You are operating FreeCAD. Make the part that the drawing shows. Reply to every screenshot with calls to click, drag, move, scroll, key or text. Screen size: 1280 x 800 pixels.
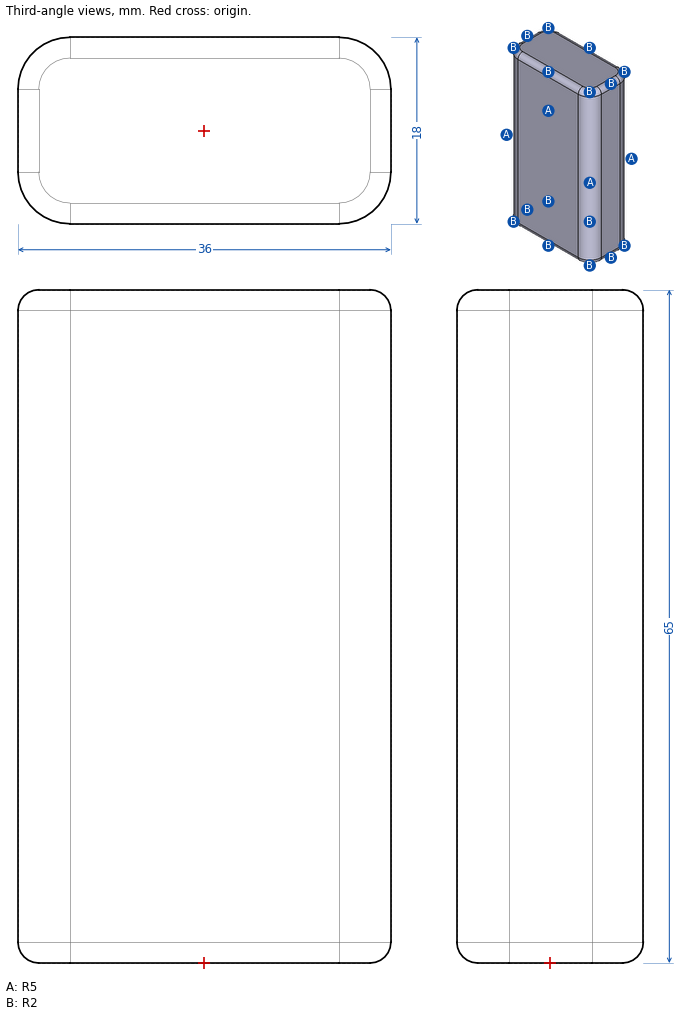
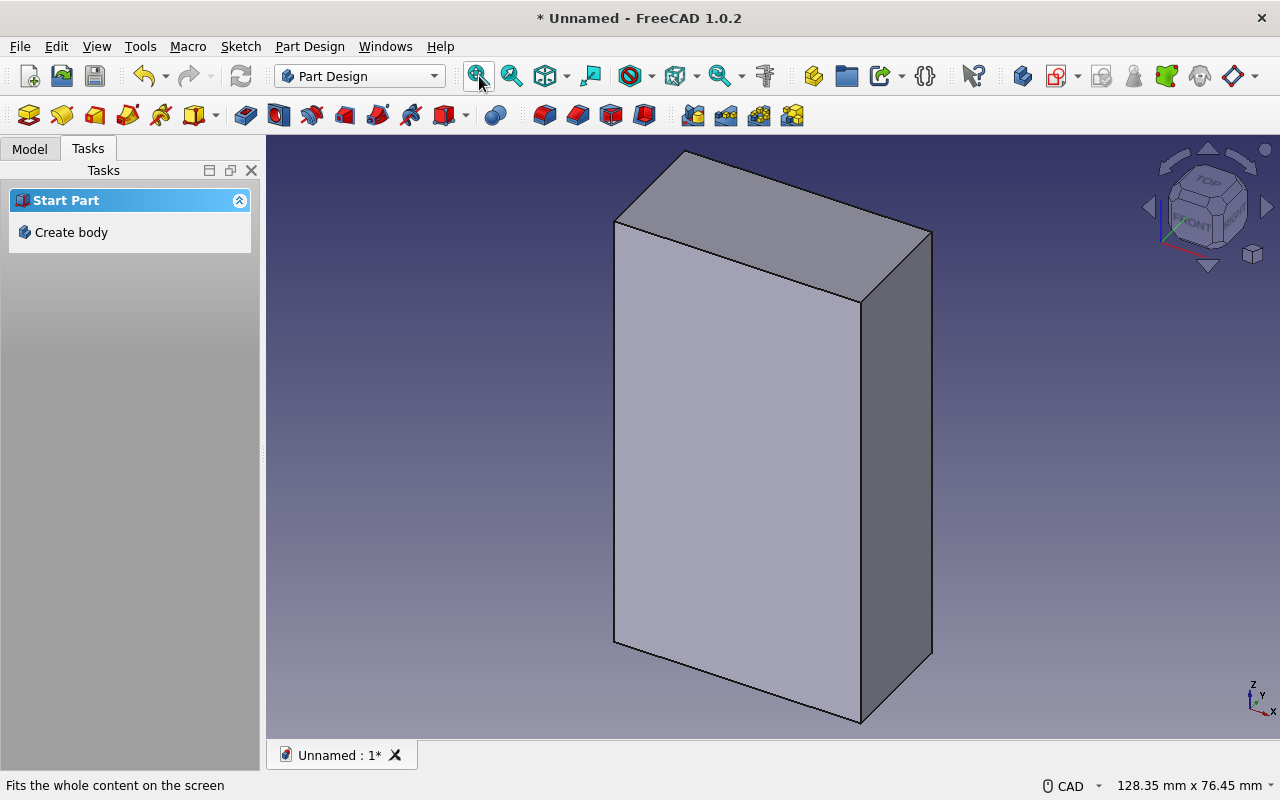
click(861, 512)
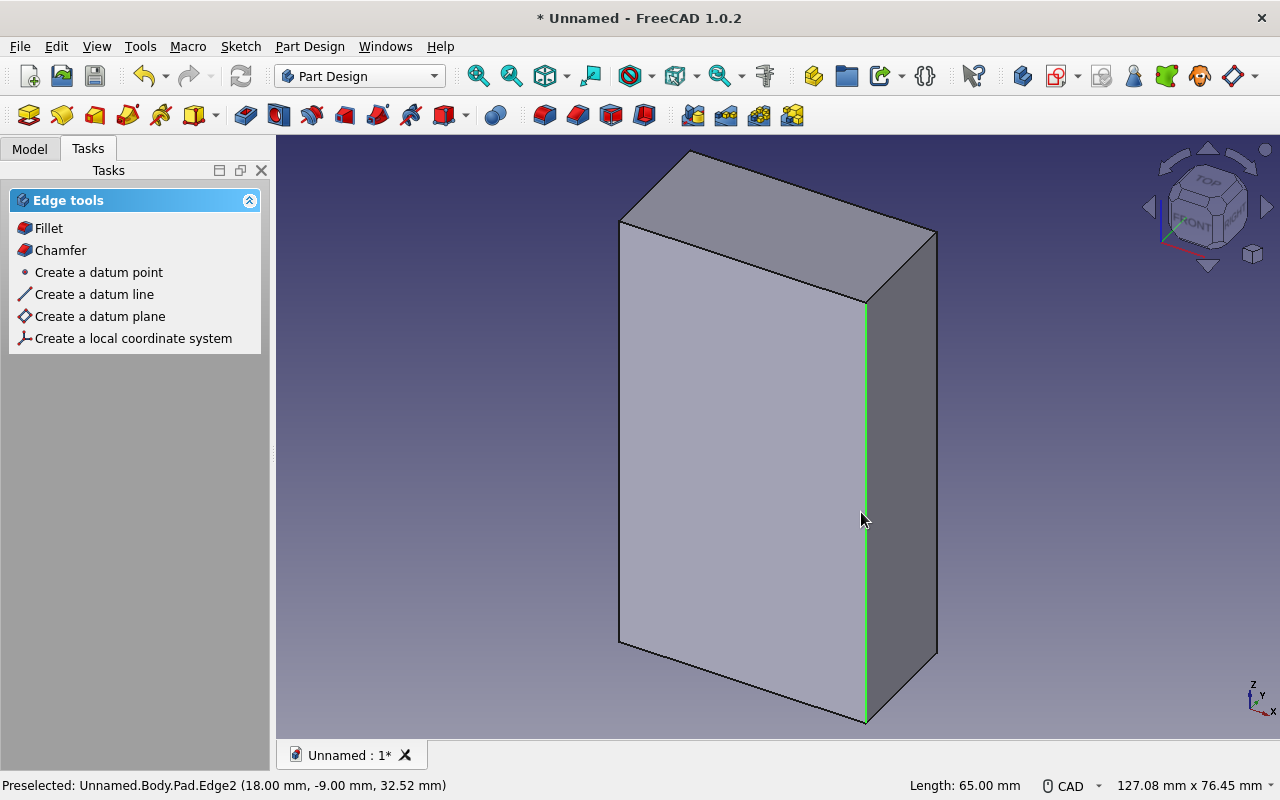
key(0)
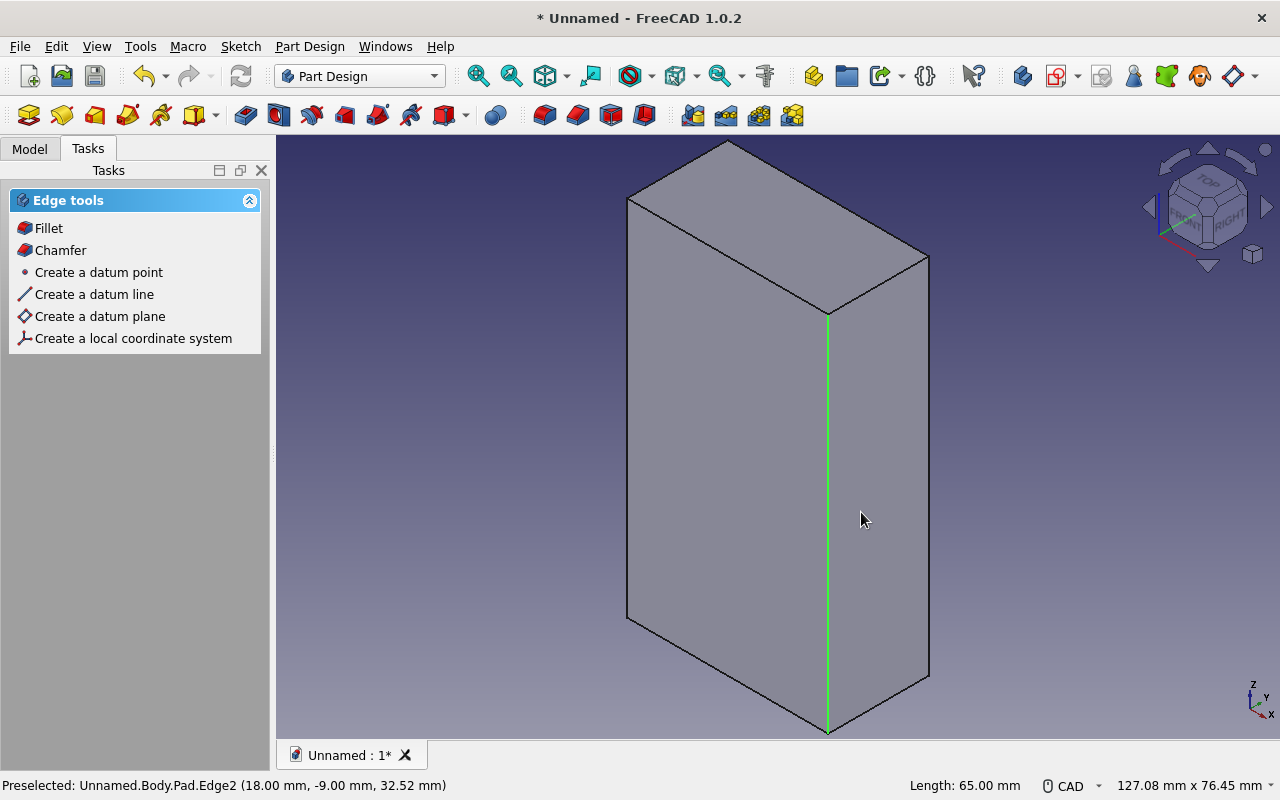
key(2)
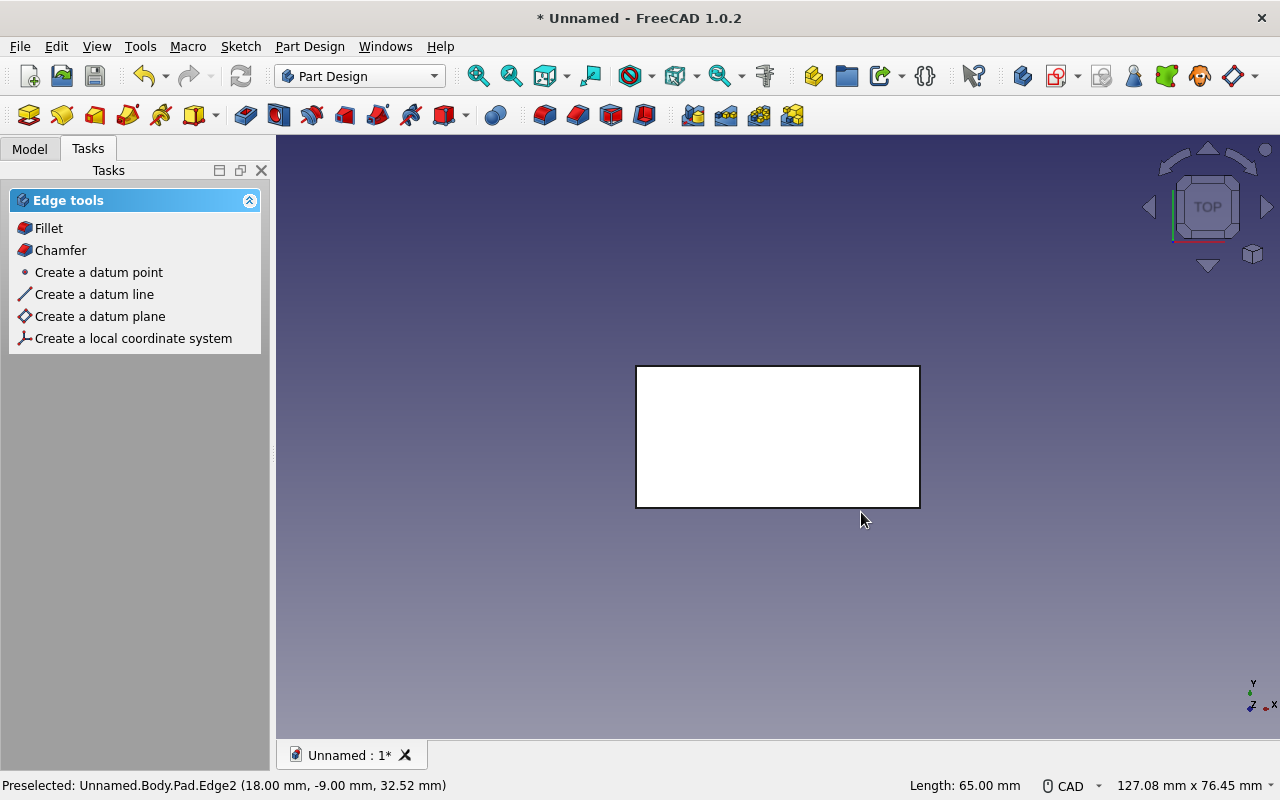
click(479, 76)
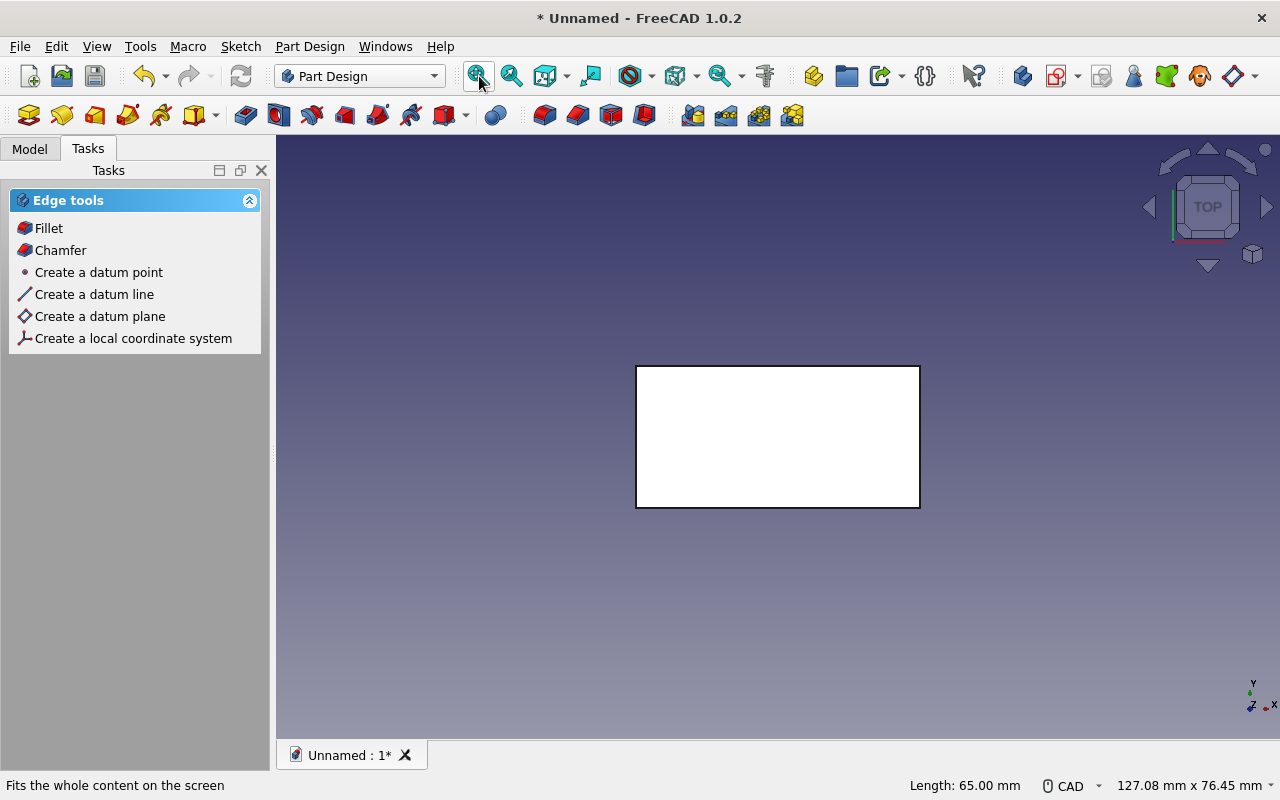
key(1)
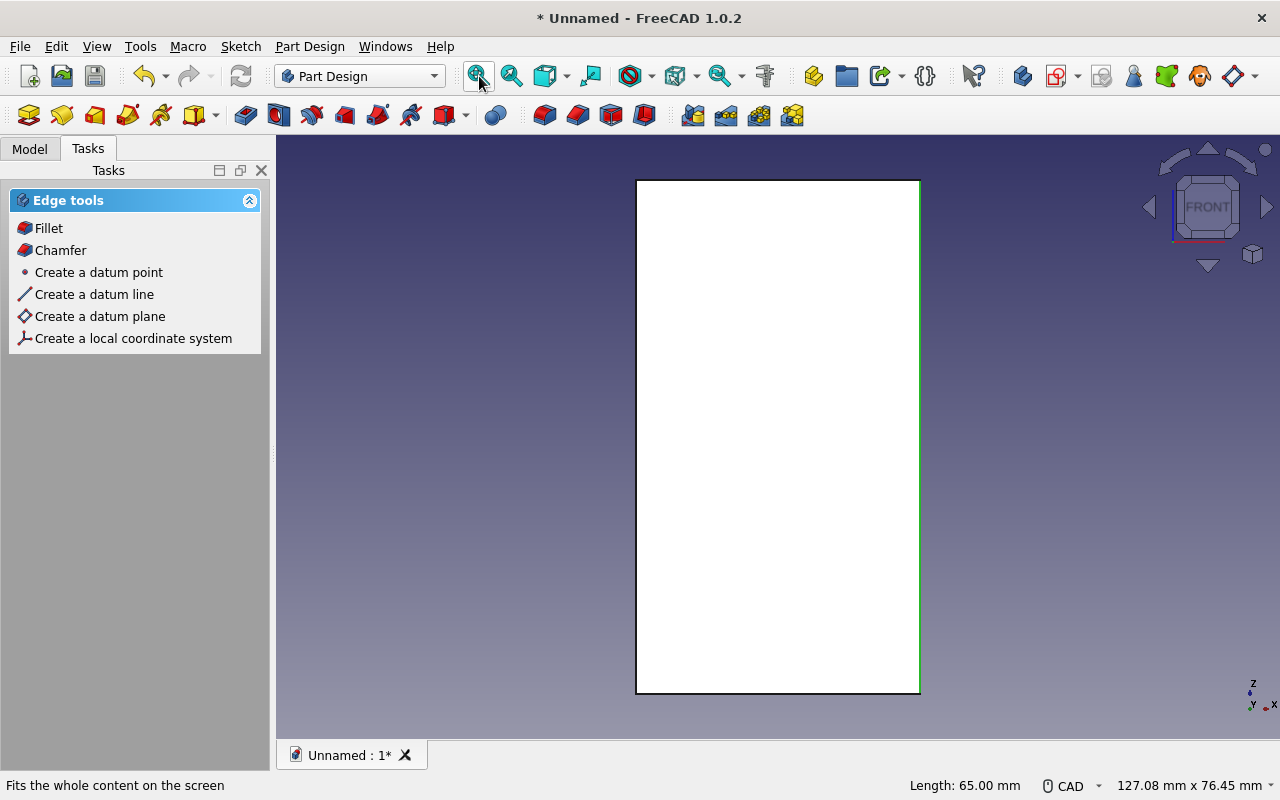
click(636, 436, ctrl)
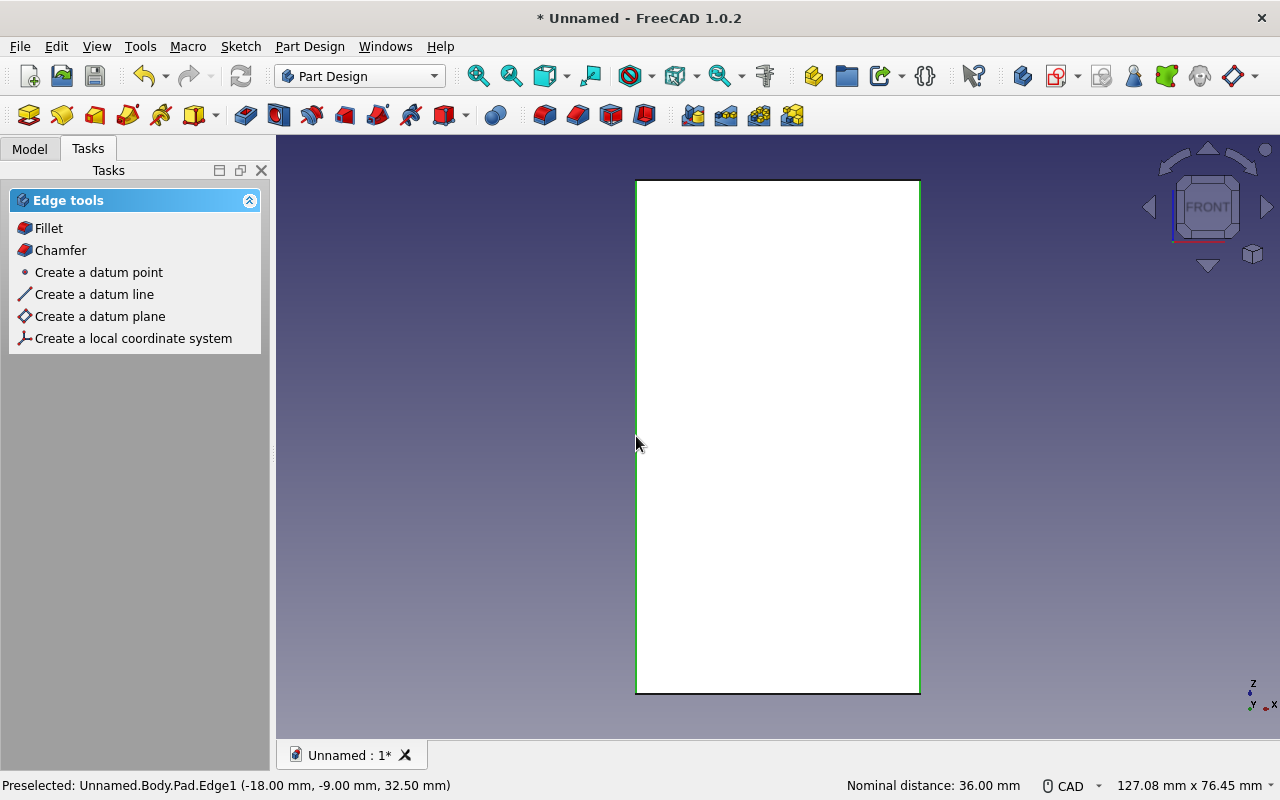
key(3)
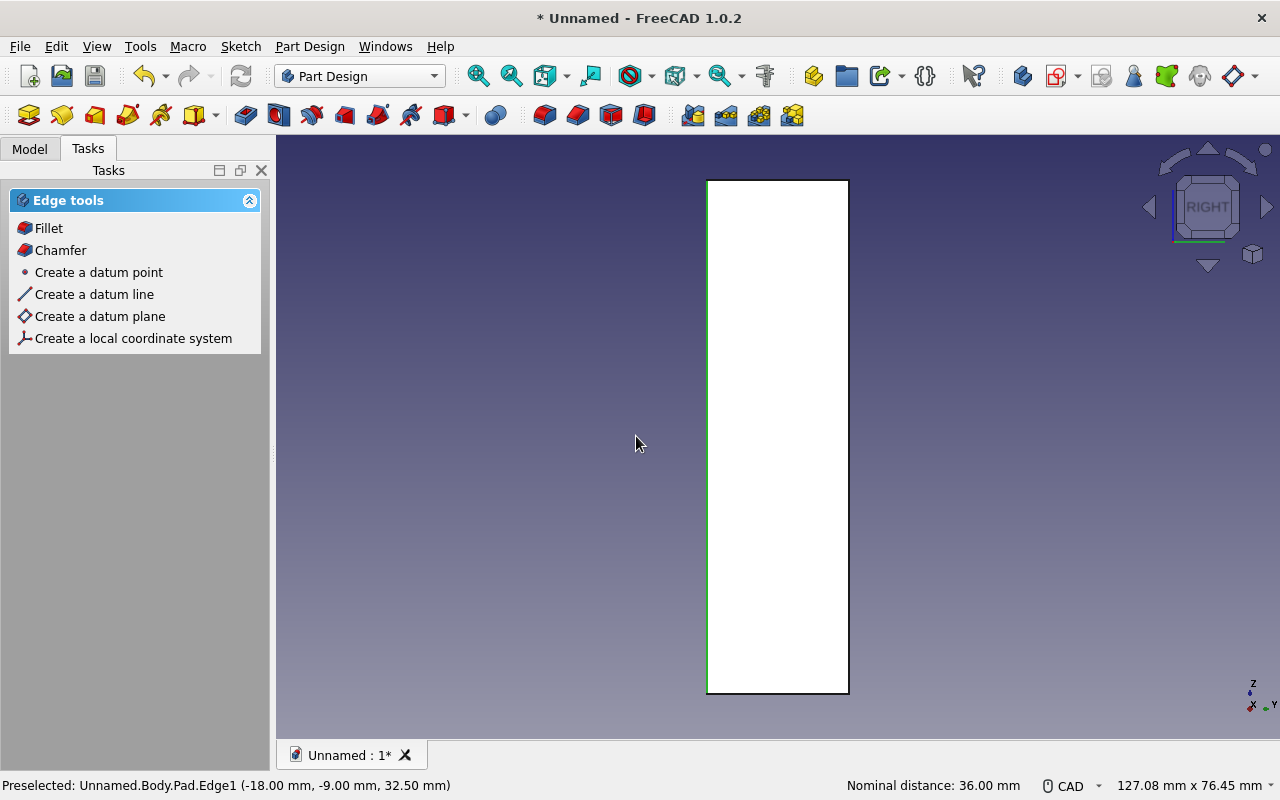
click(849, 436, ctrl)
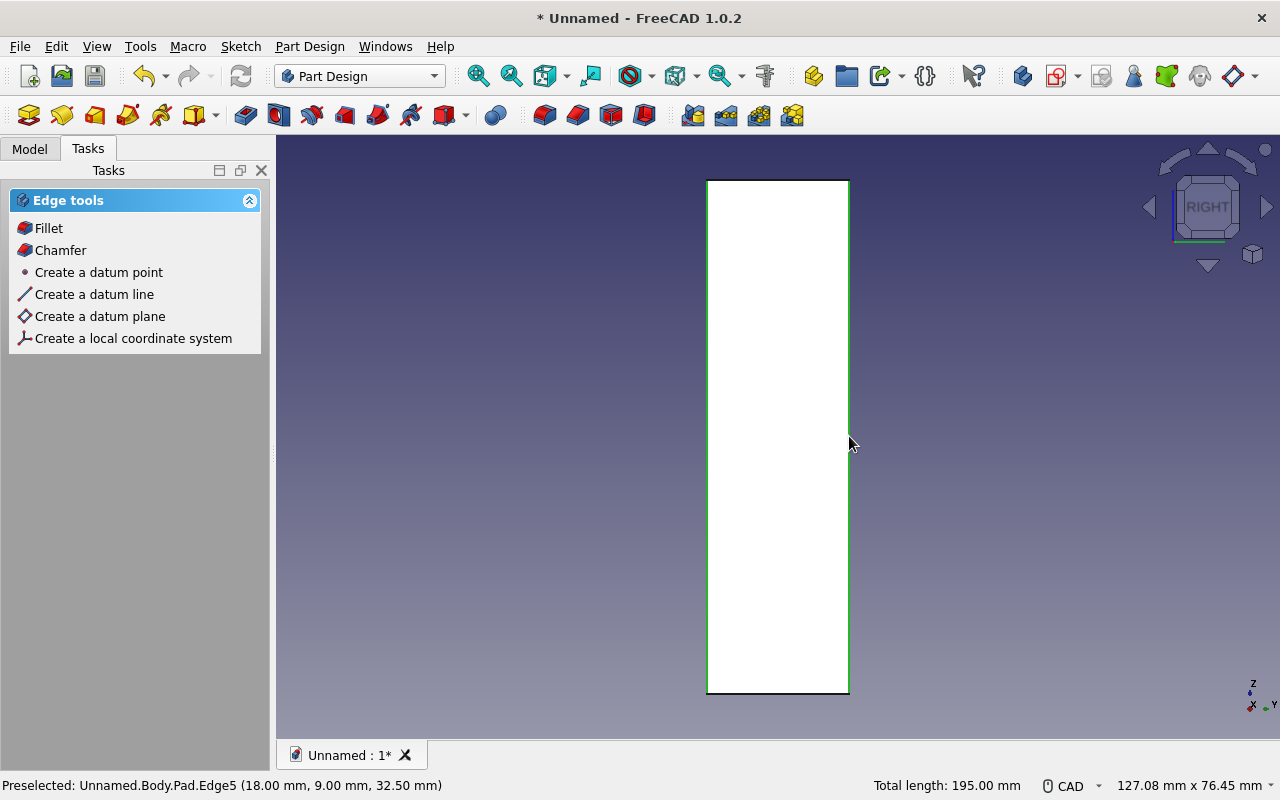
key(5)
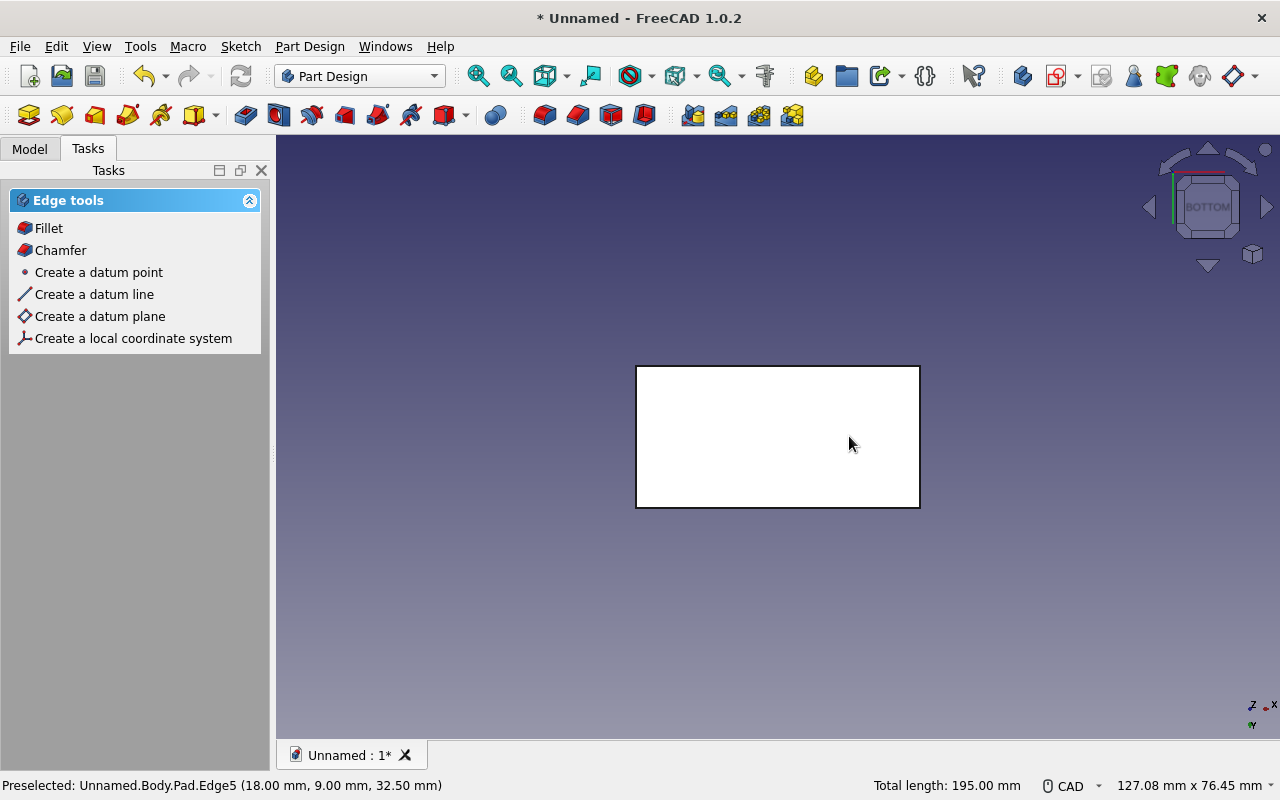
click(479, 76)